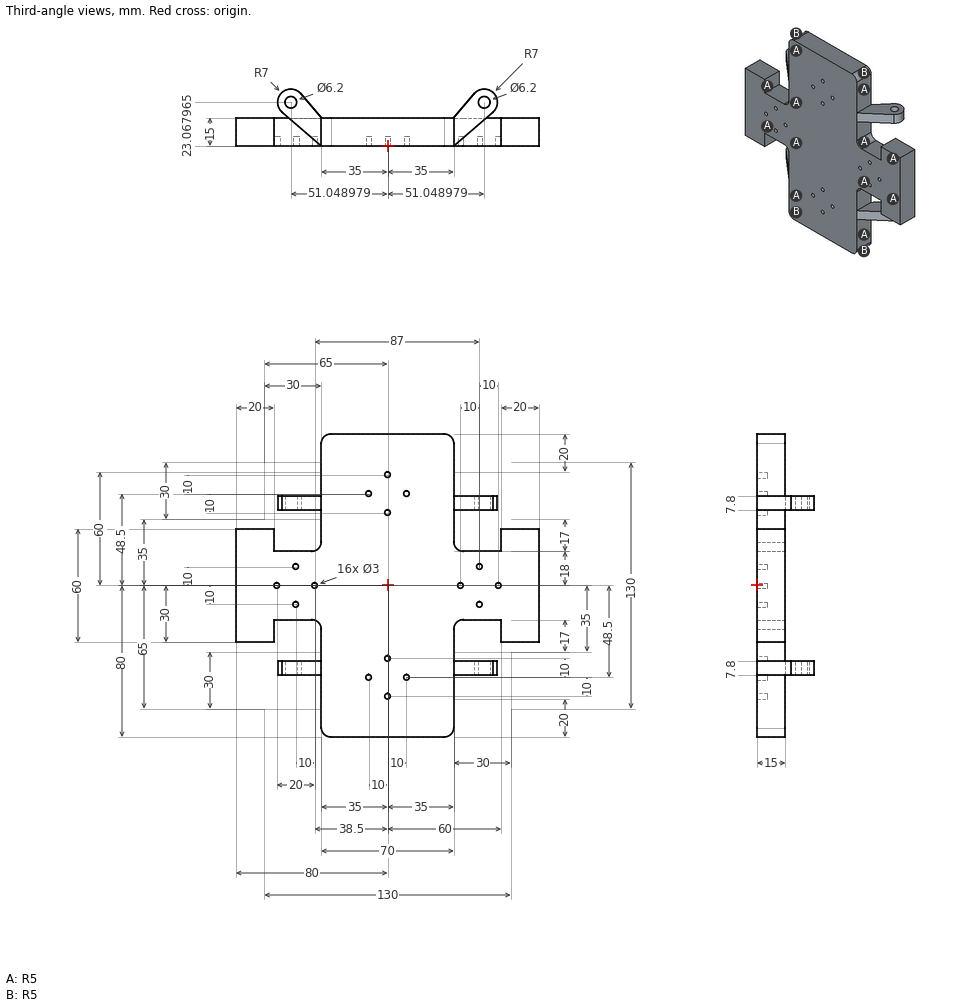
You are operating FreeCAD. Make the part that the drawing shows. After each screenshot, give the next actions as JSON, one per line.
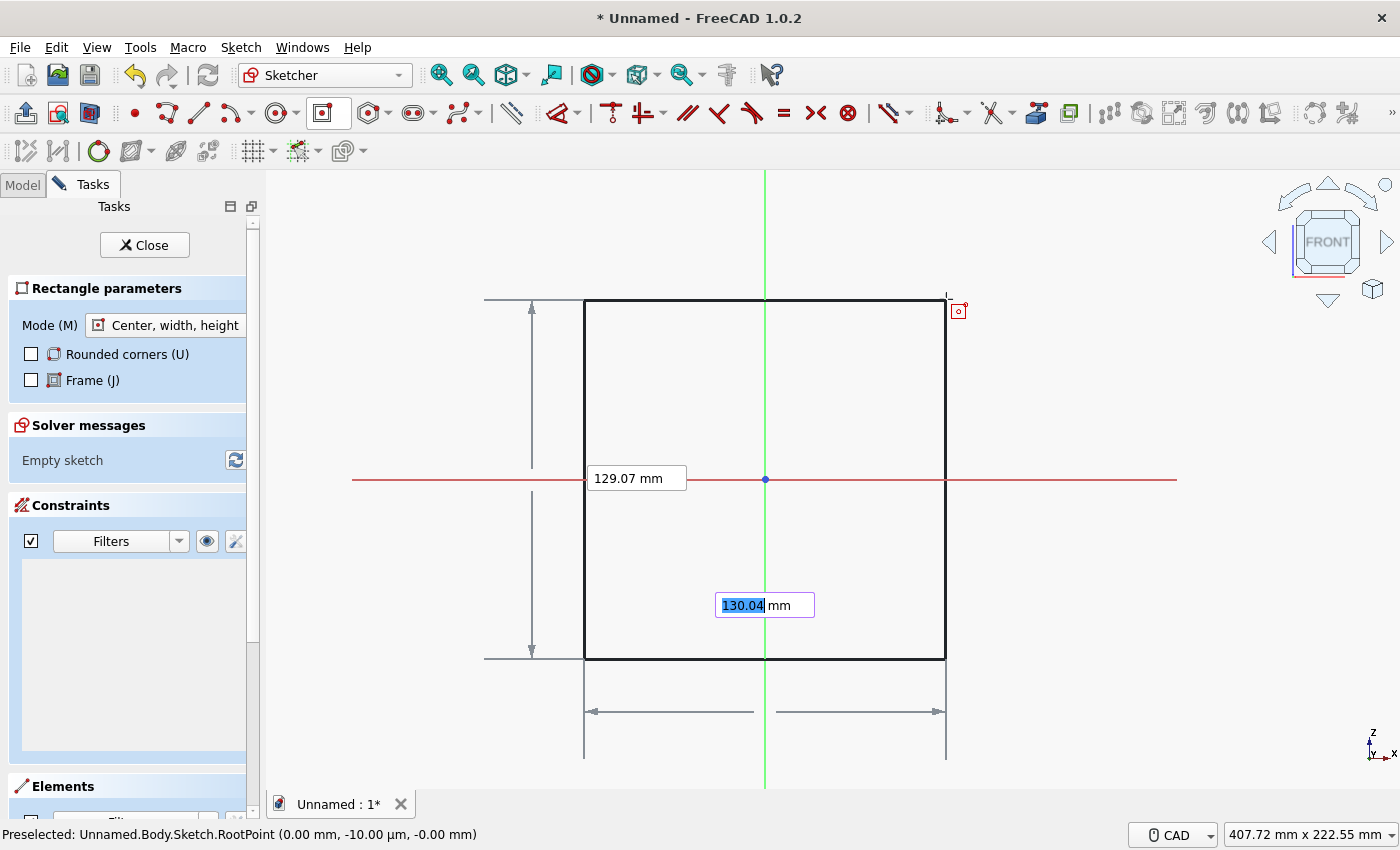
{"action": "type", "text": "130"}
{"action": "key", "text": "Tab"}
{"action": "type", "text": "130"}
{"action": "key", "text": "Return"}
{"action": "key", "text": "Escape"}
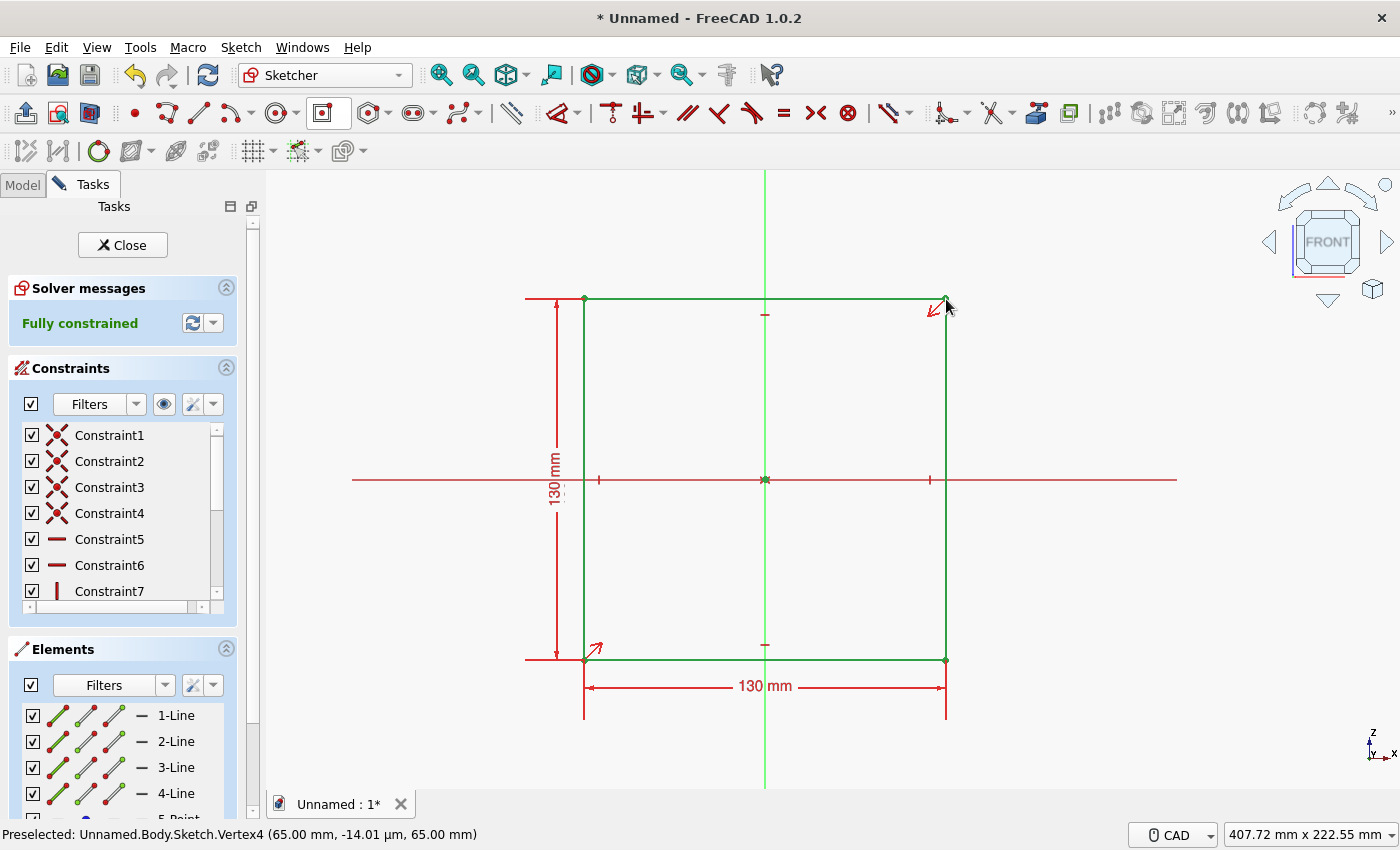
{"action": "left_click", "coordinate": [123, 245]}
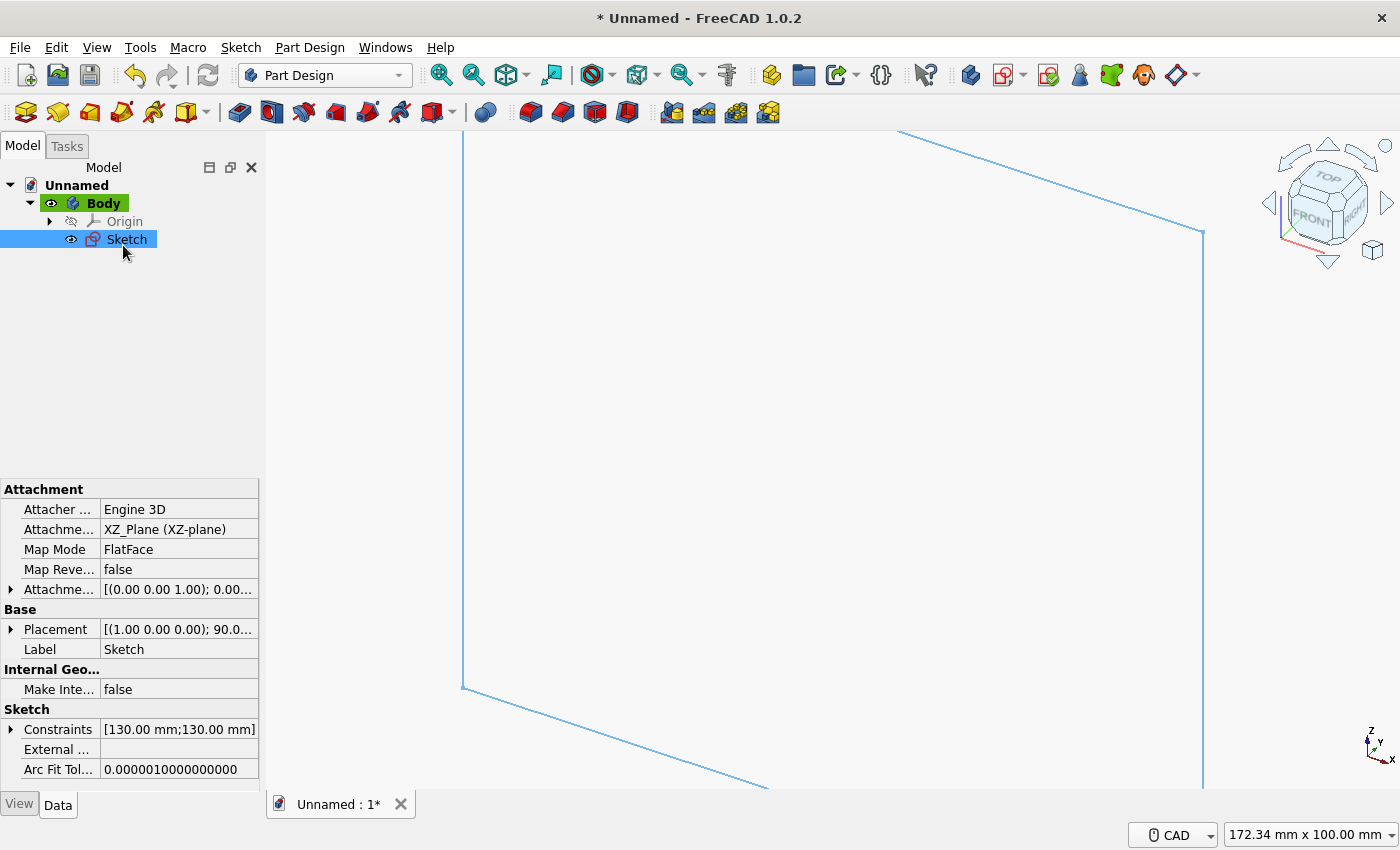
{"action": "left_click", "coordinate": [26, 112]}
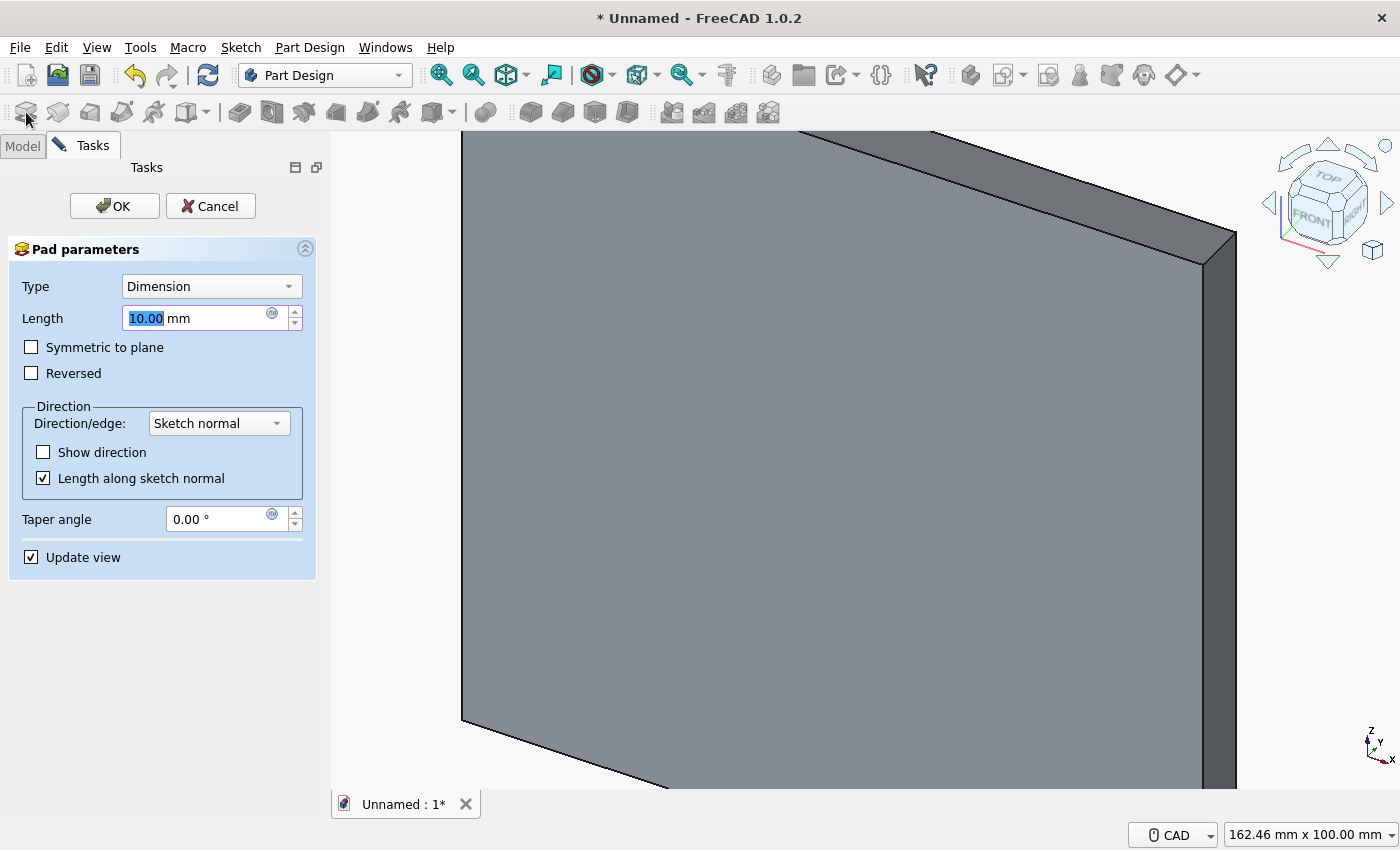
{"action": "type", "text": "15"}
{"action": "key", "text": "Tab"}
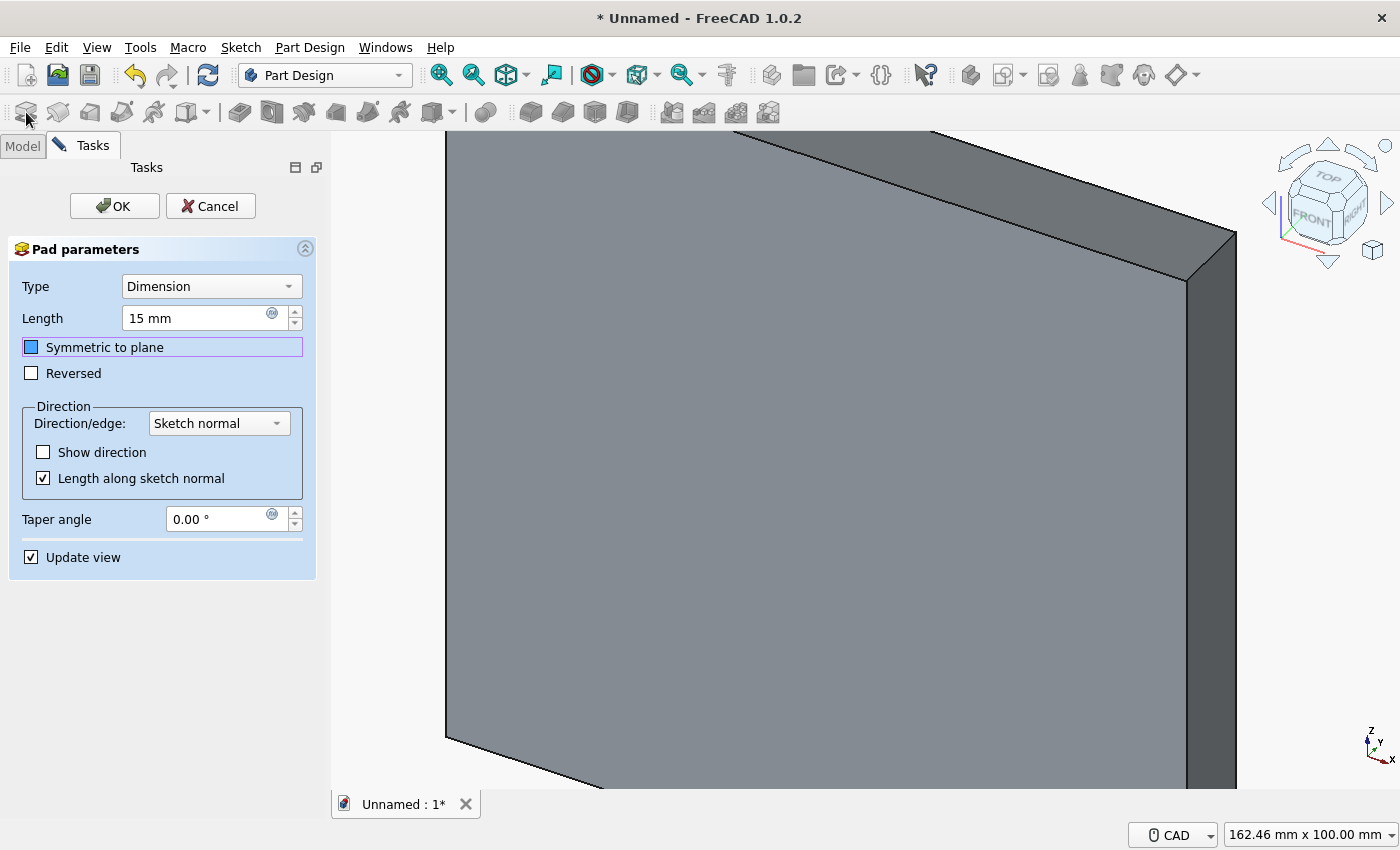
{"action": "left_click", "coordinate": [30, 373]}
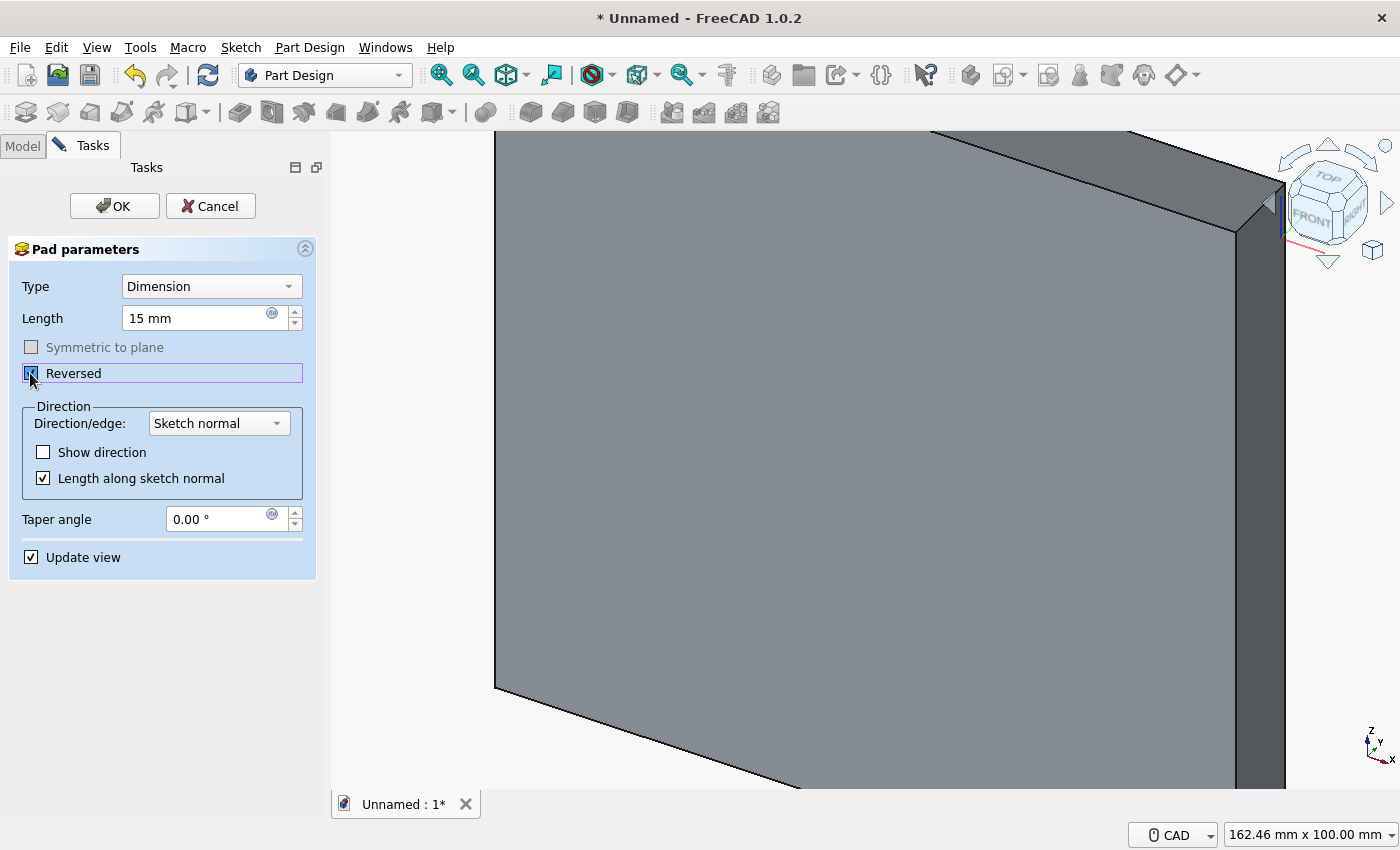
{"action": "left_click", "coordinate": [115, 206]}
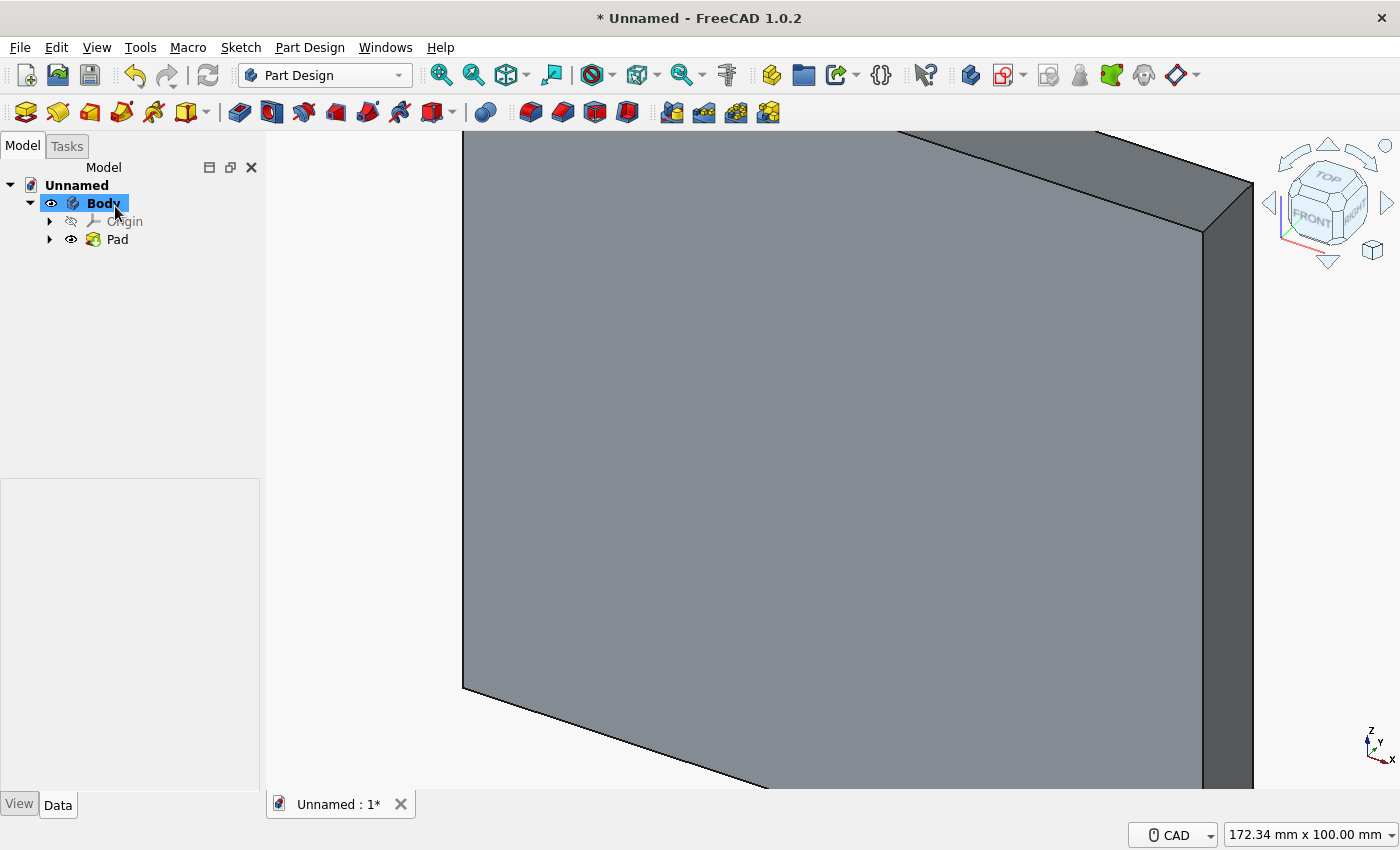
{"action": "left_click", "coordinate": [442, 76]}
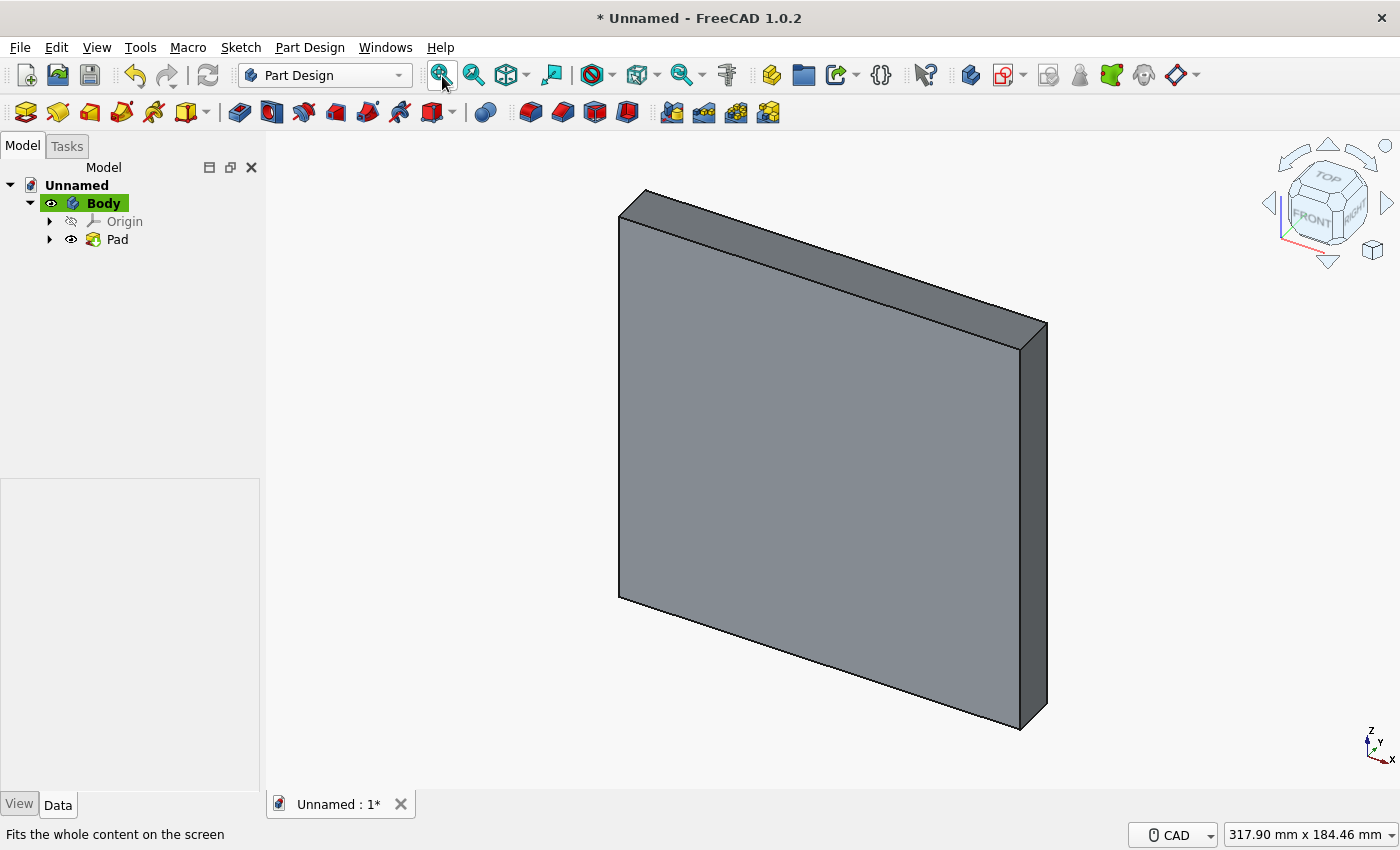
{"action": "key", "text": "4"}